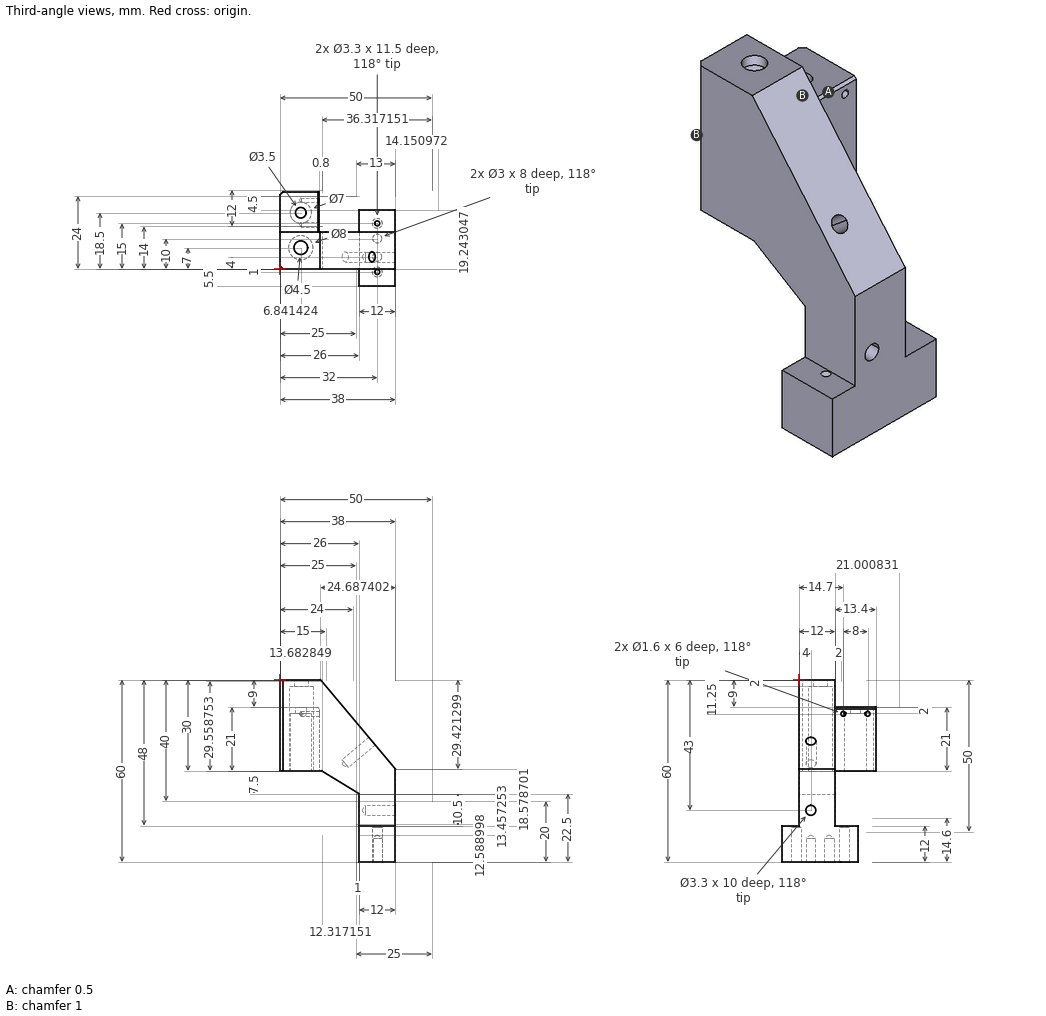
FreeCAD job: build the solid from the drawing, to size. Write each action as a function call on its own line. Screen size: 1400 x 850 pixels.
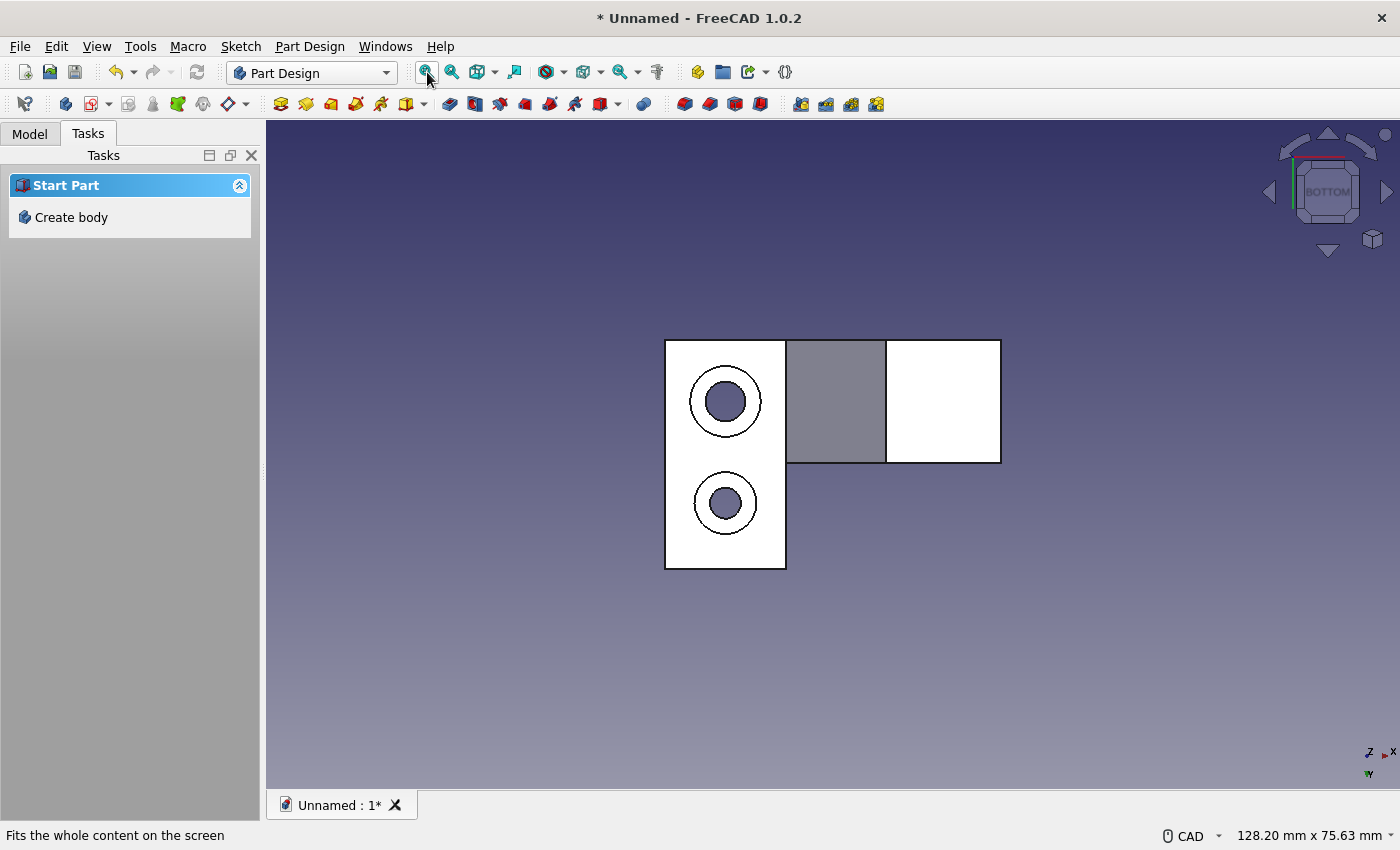
click(944, 400)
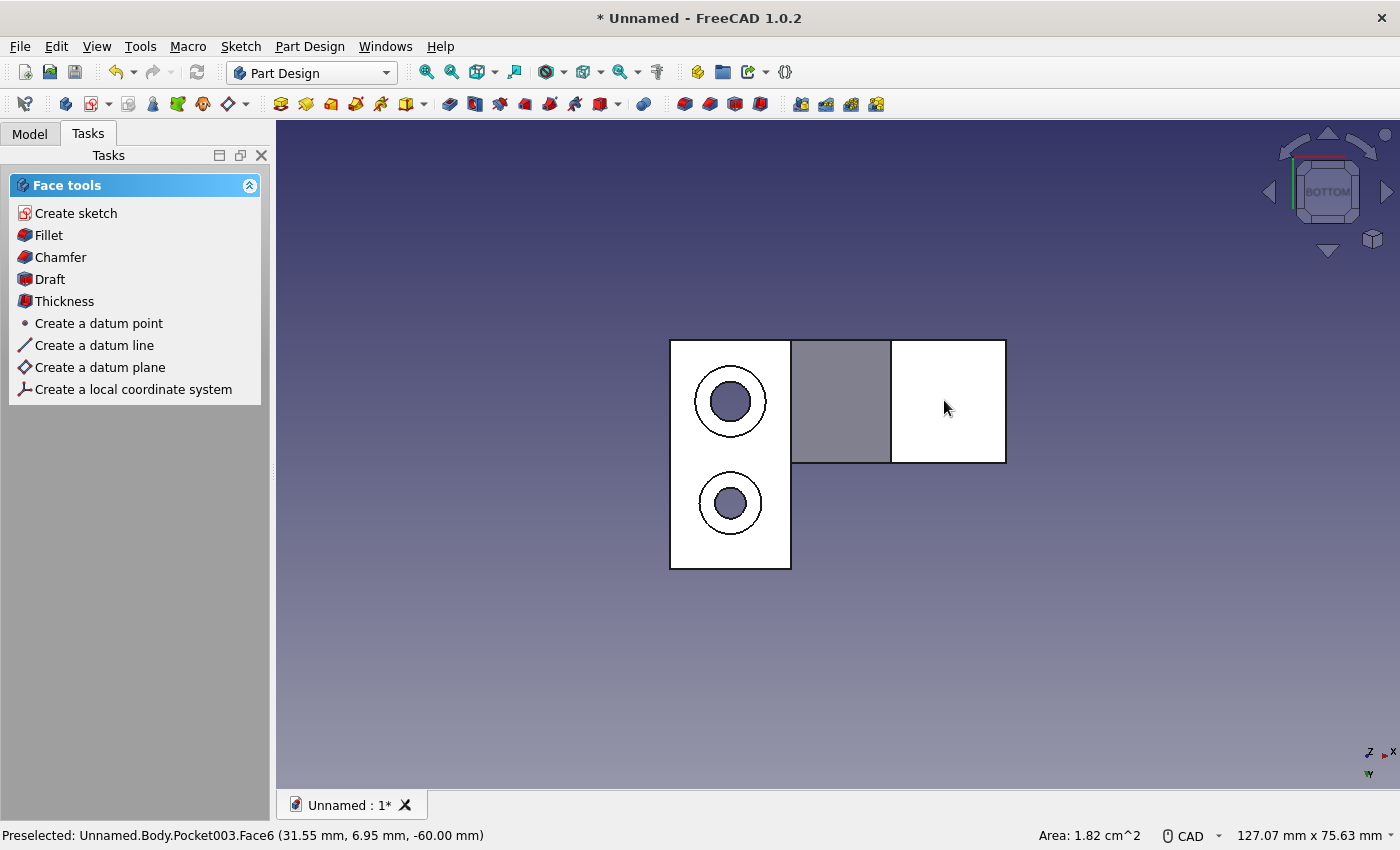
click(90, 104)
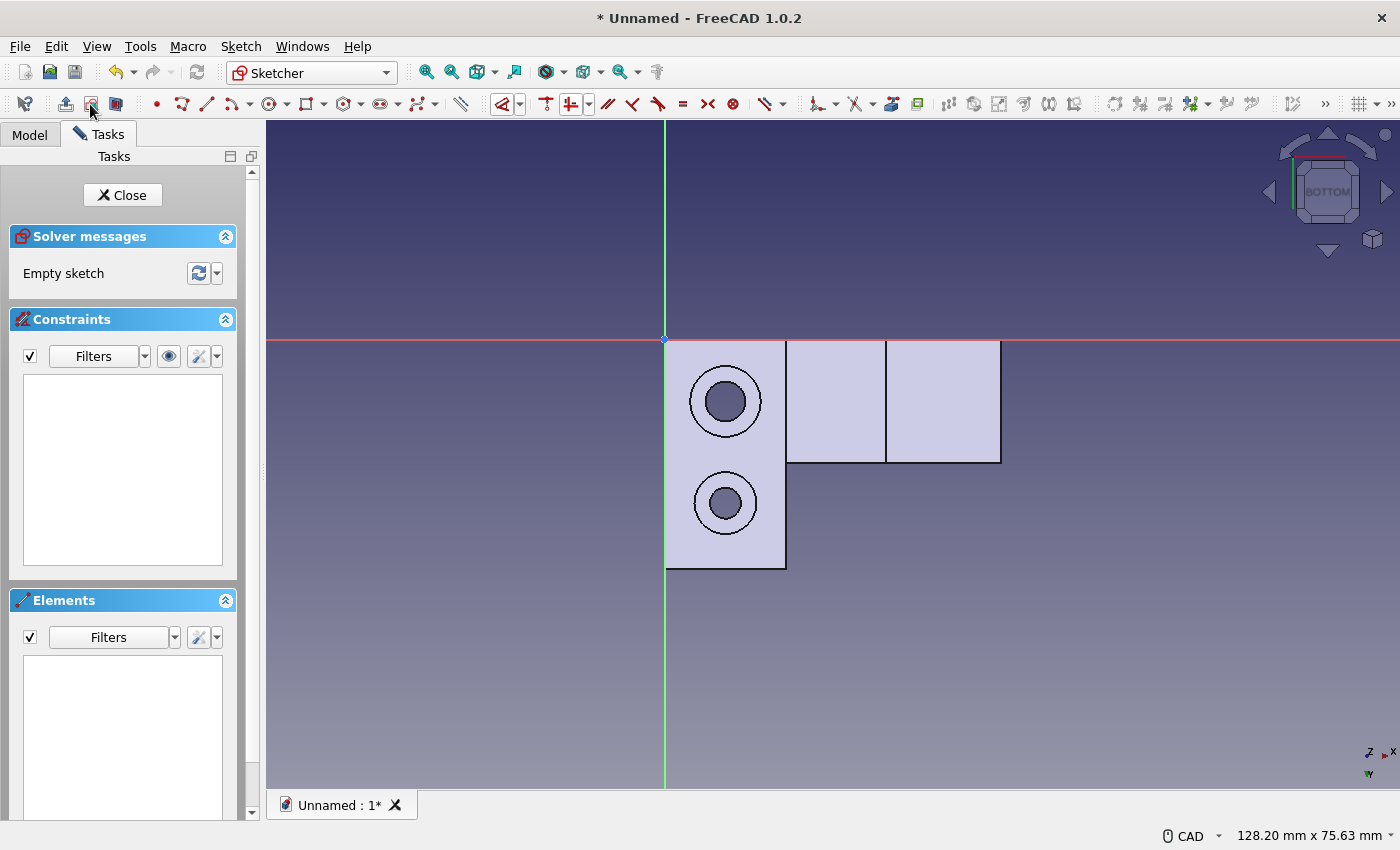
scroll(916, 435, up, 3)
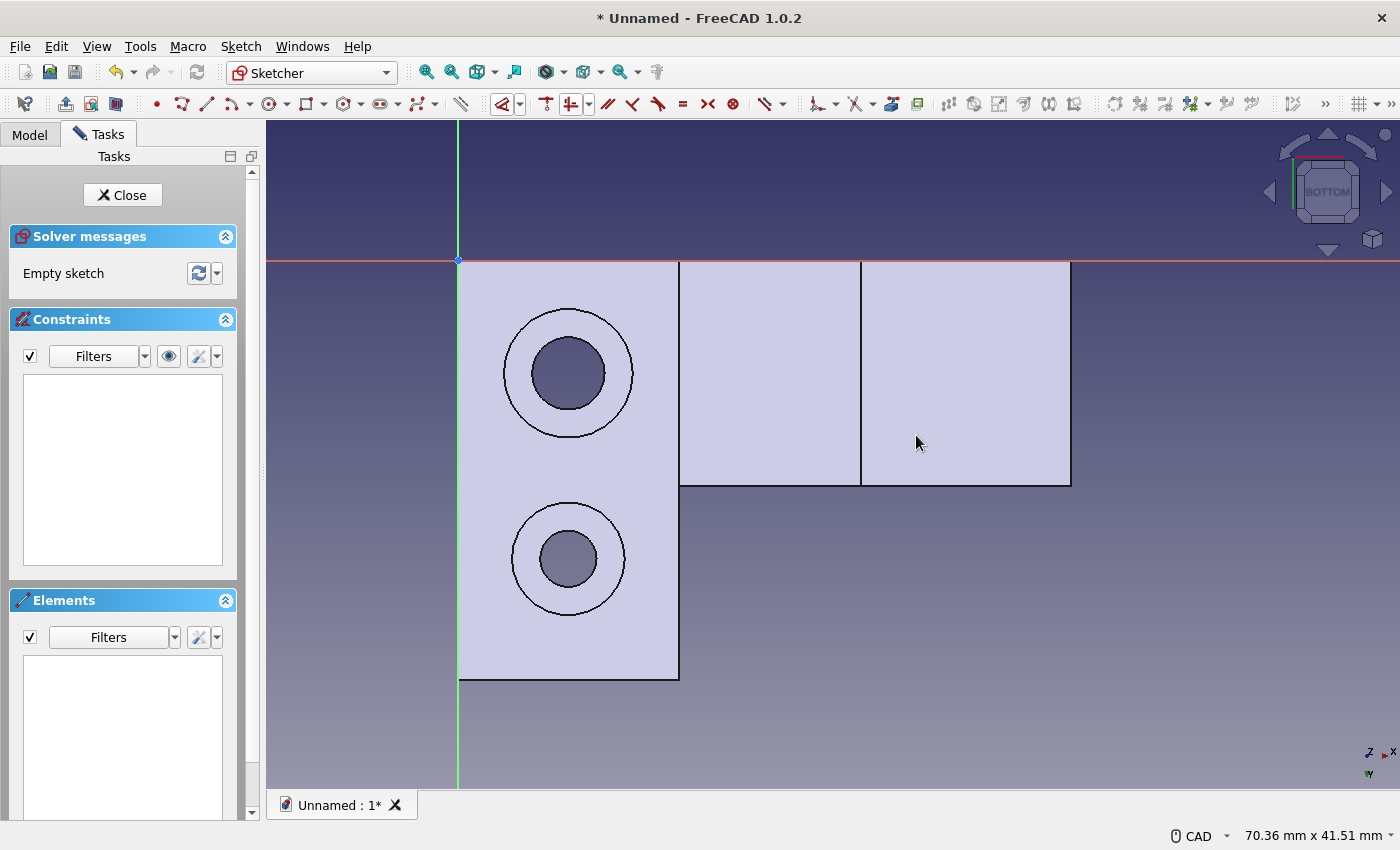
click(306, 104)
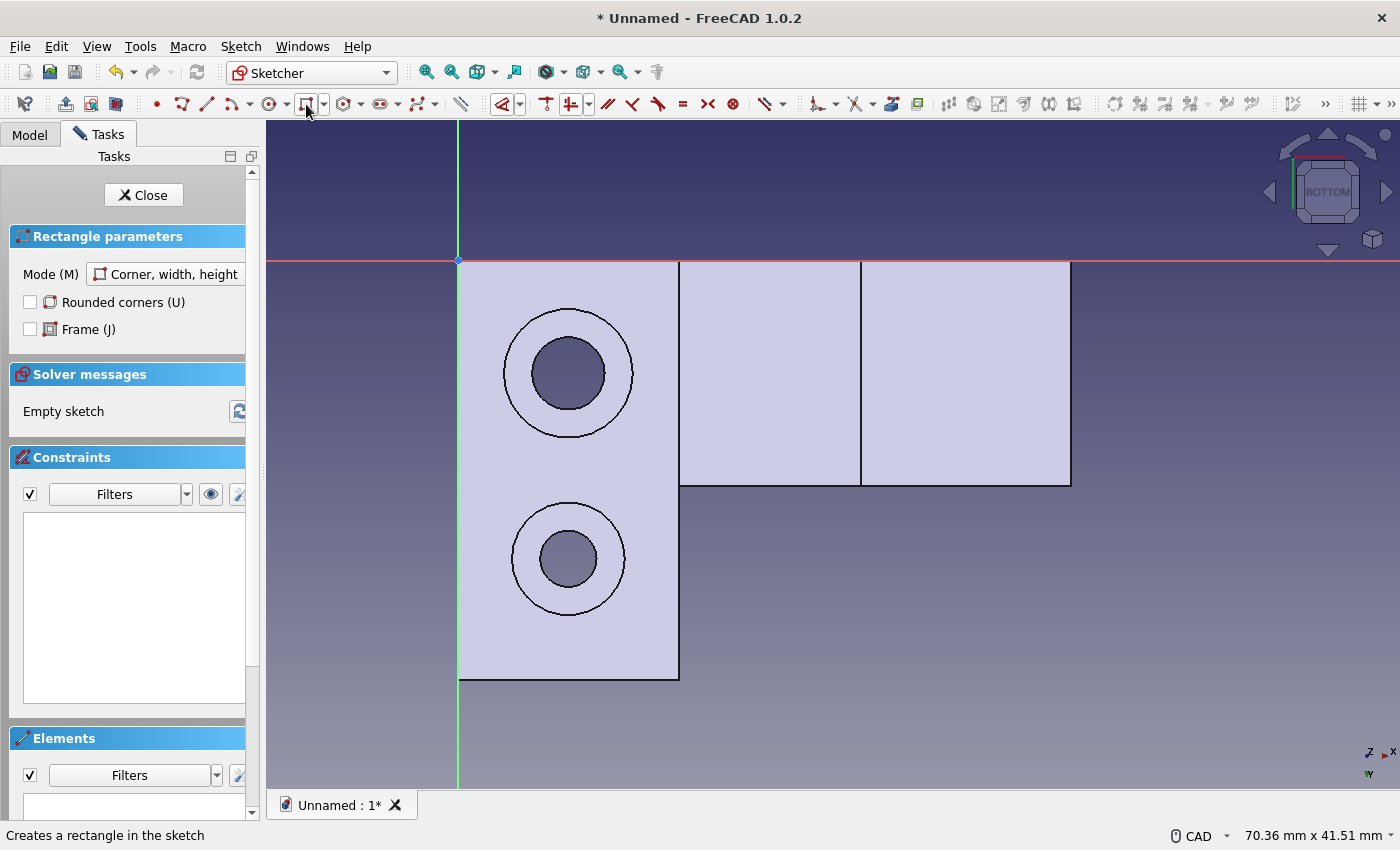
click(861, 261)
click(1071, 647)
key(Escape)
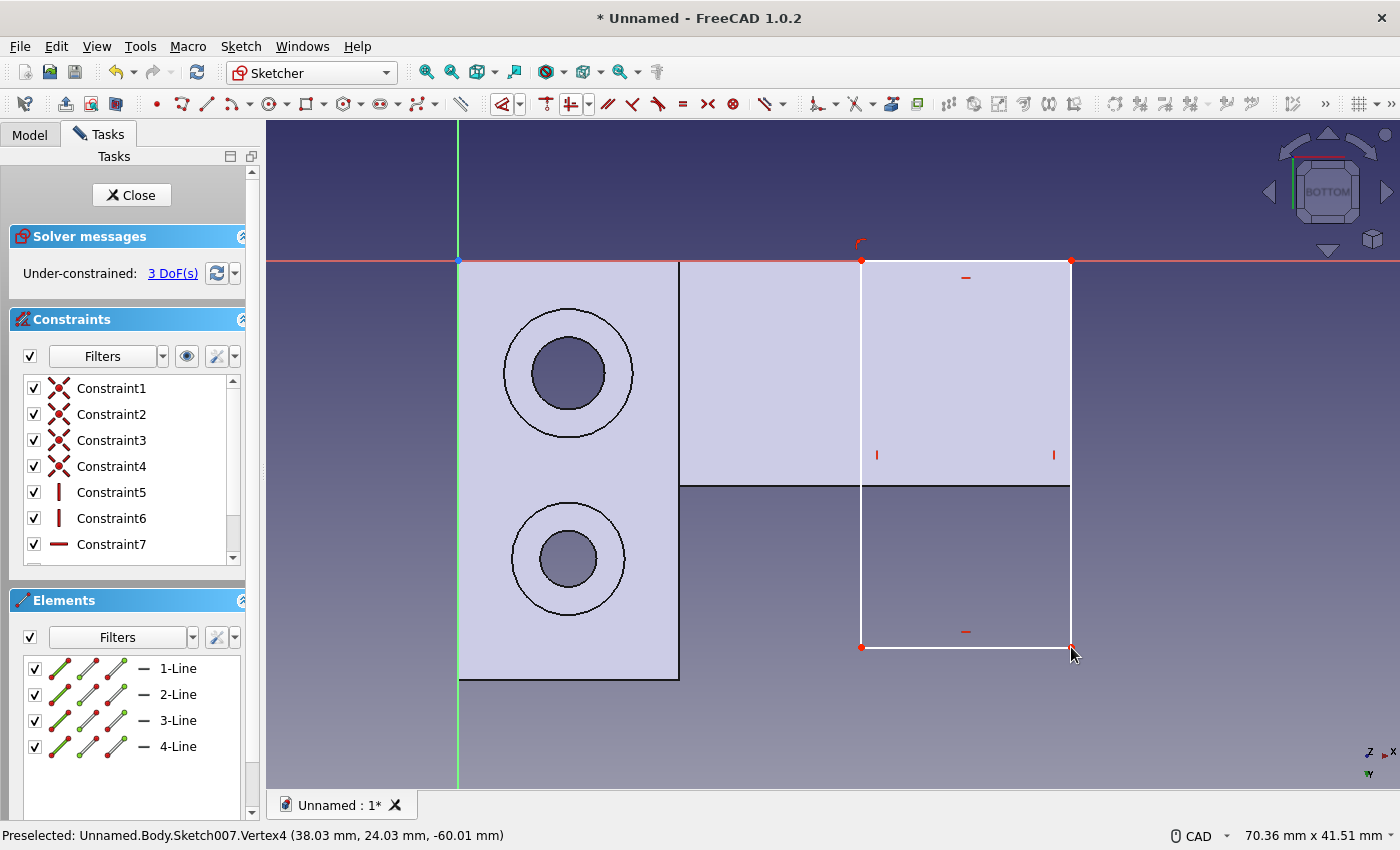
click(861, 377)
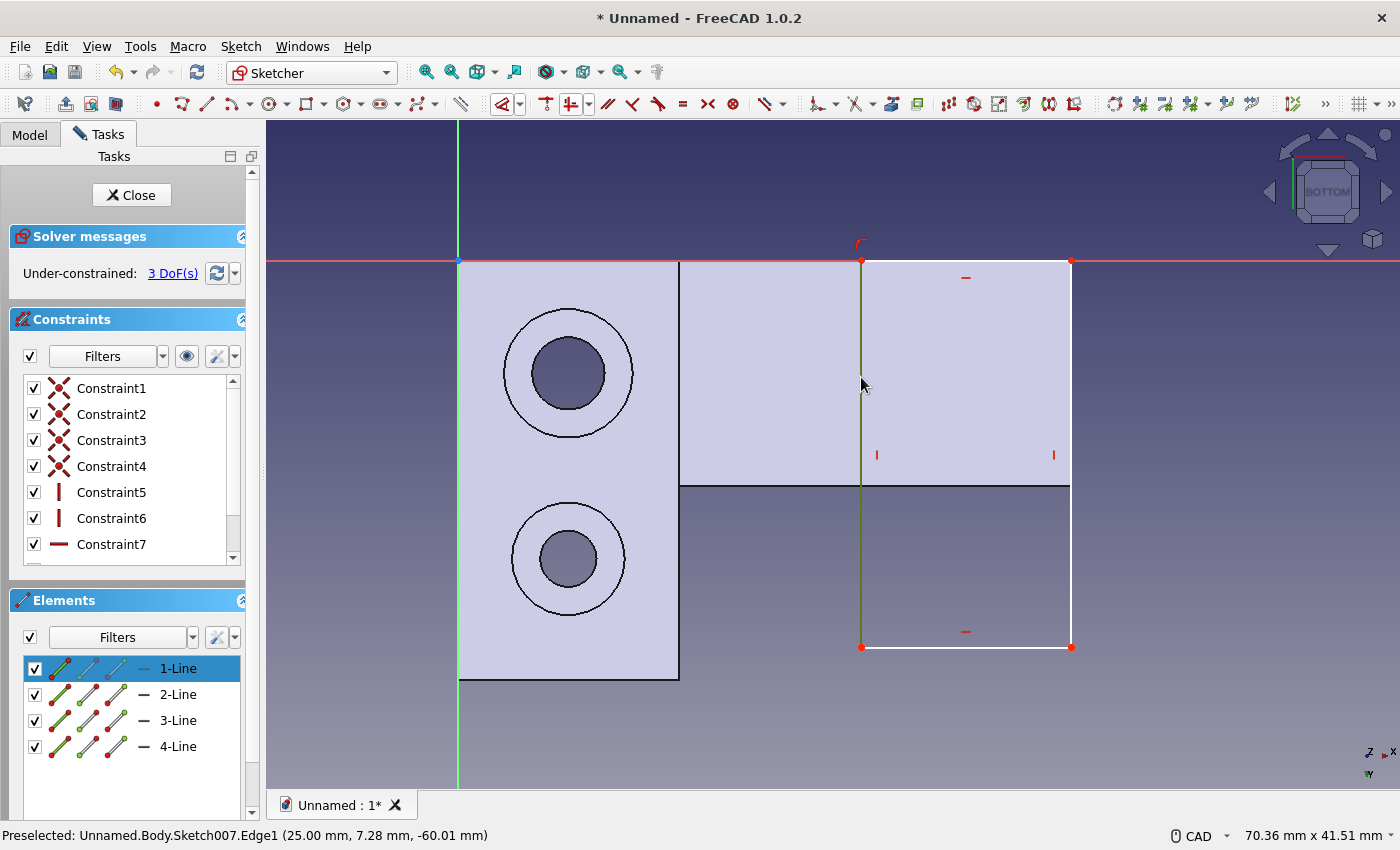
click(520, 104)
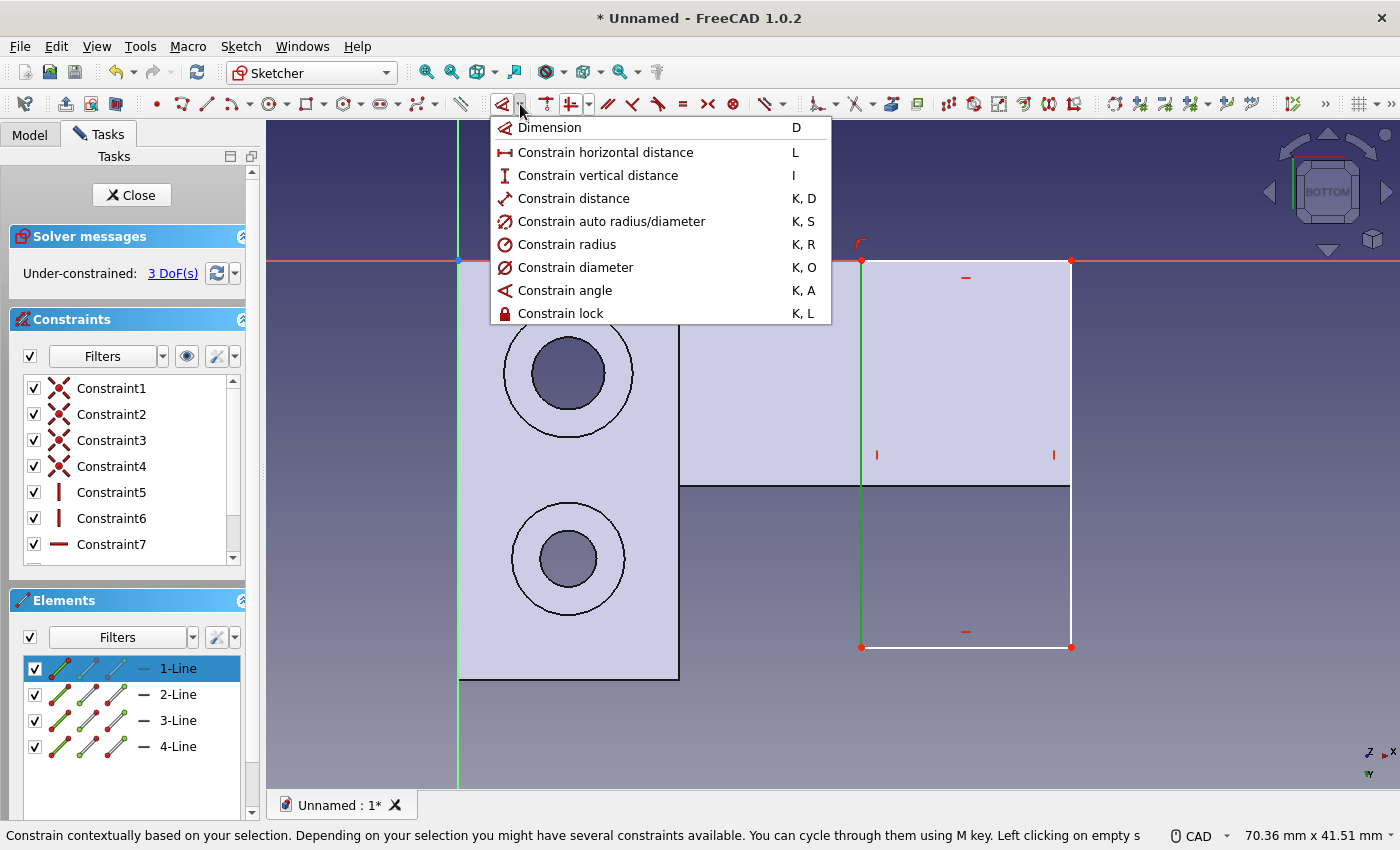
click(661, 176)